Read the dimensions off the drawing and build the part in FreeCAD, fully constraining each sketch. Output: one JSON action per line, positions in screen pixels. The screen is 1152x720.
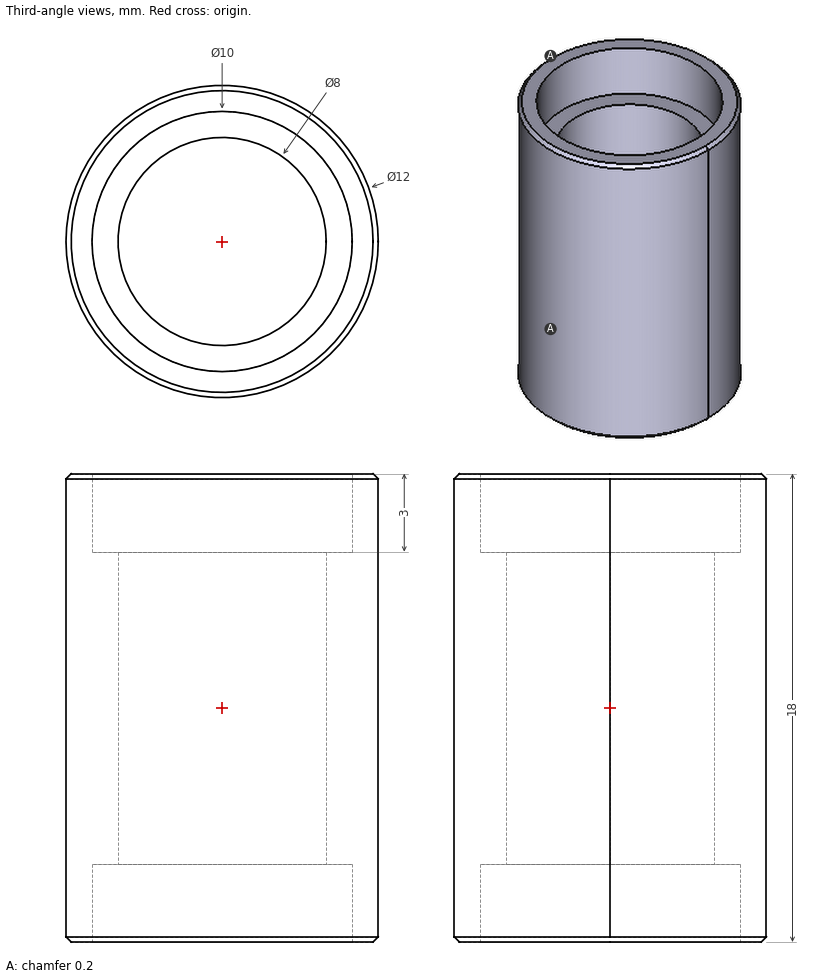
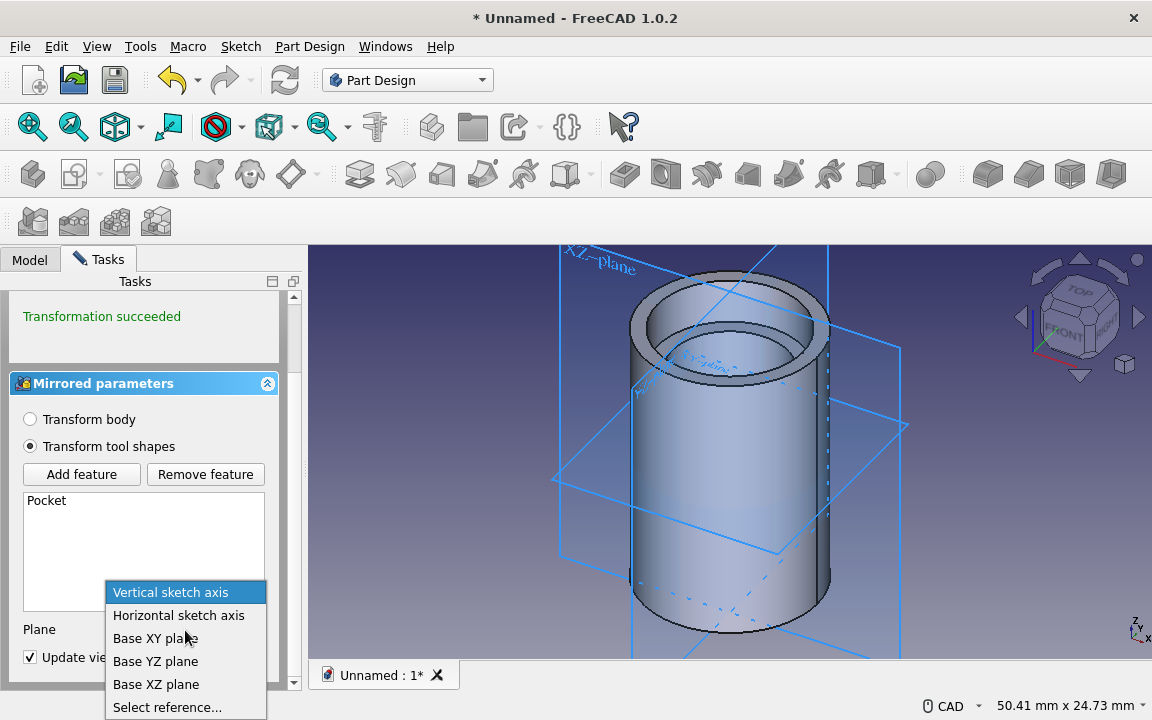
{"action": "left_click", "coordinate": [184, 638]}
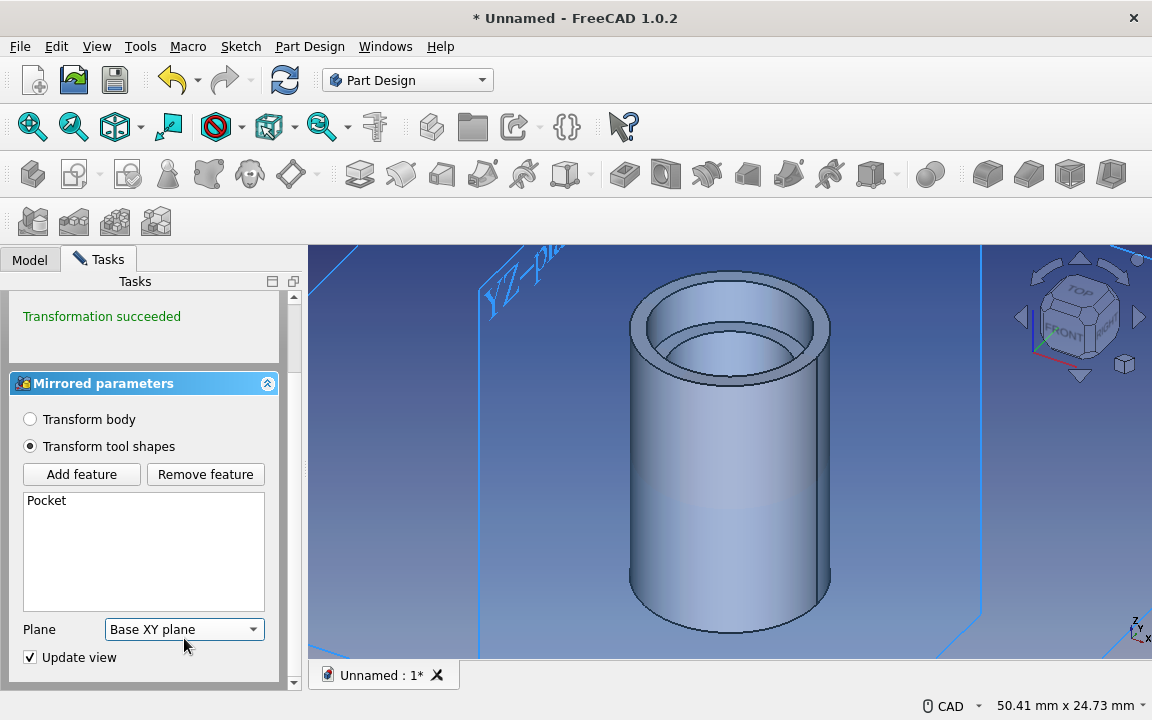
{"action": "scroll", "coordinate": [294, 490], "scroll_direction": "up", "scroll_amount": 3}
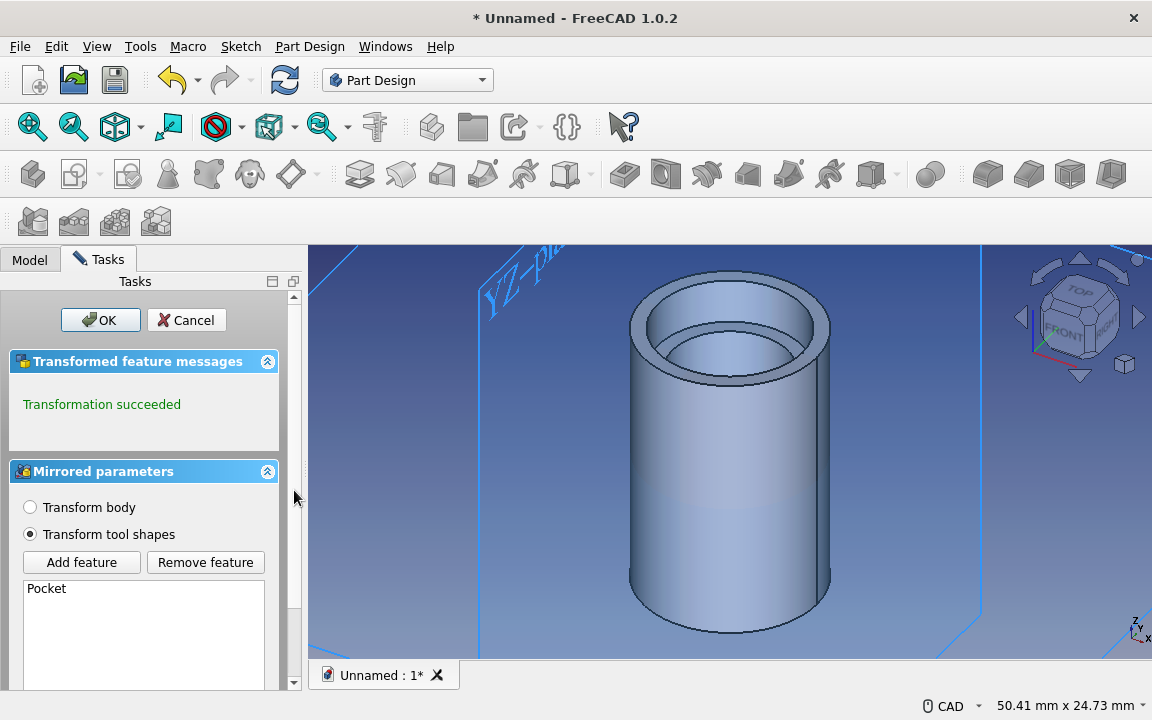
{"action": "left_click", "coordinate": [101, 320]}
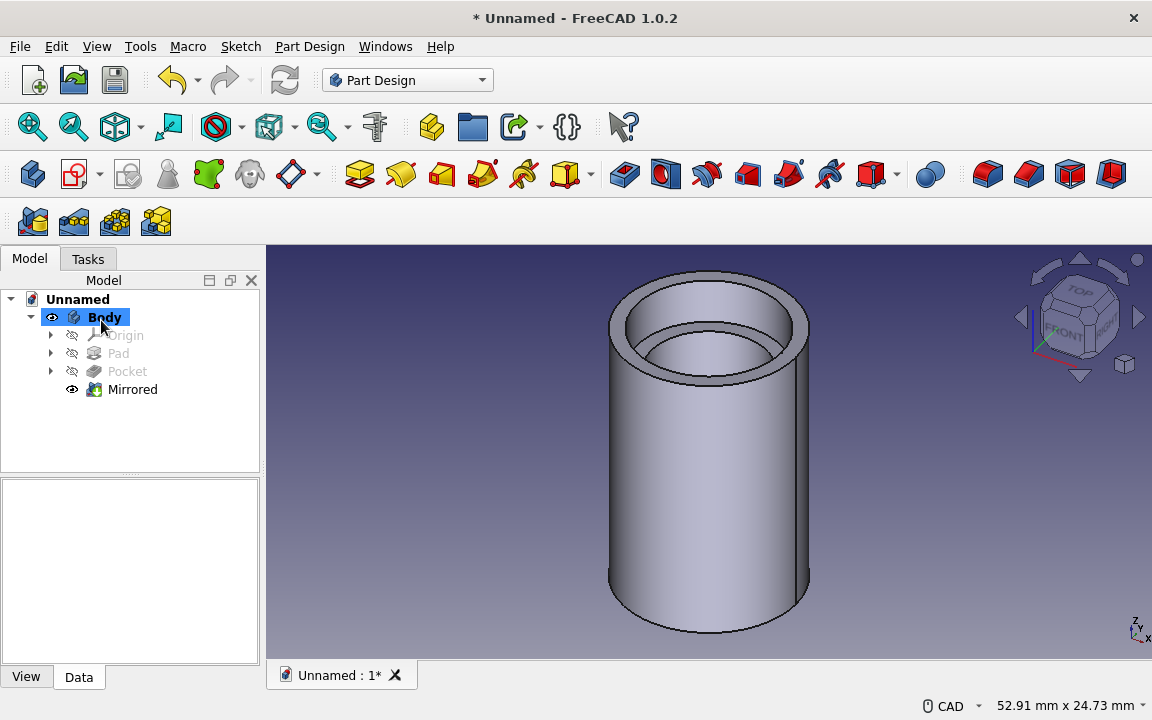
{"action": "left_click", "coordinate": [609, 334]}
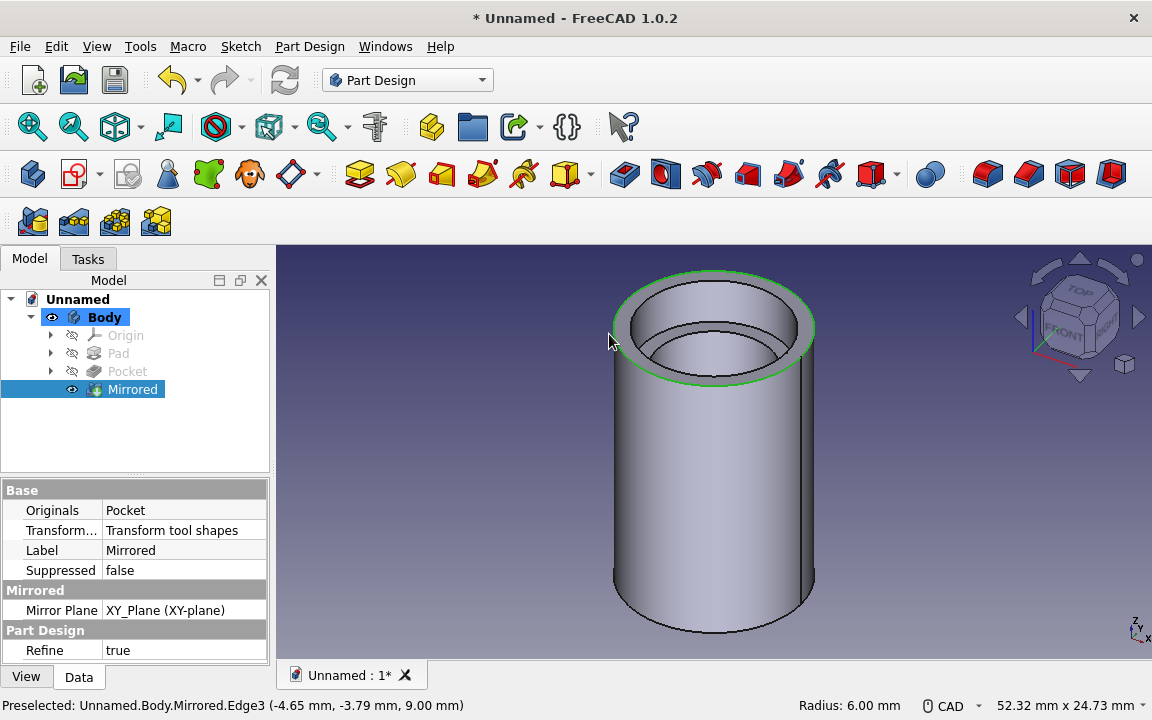
{"action": "key", "text": "0"}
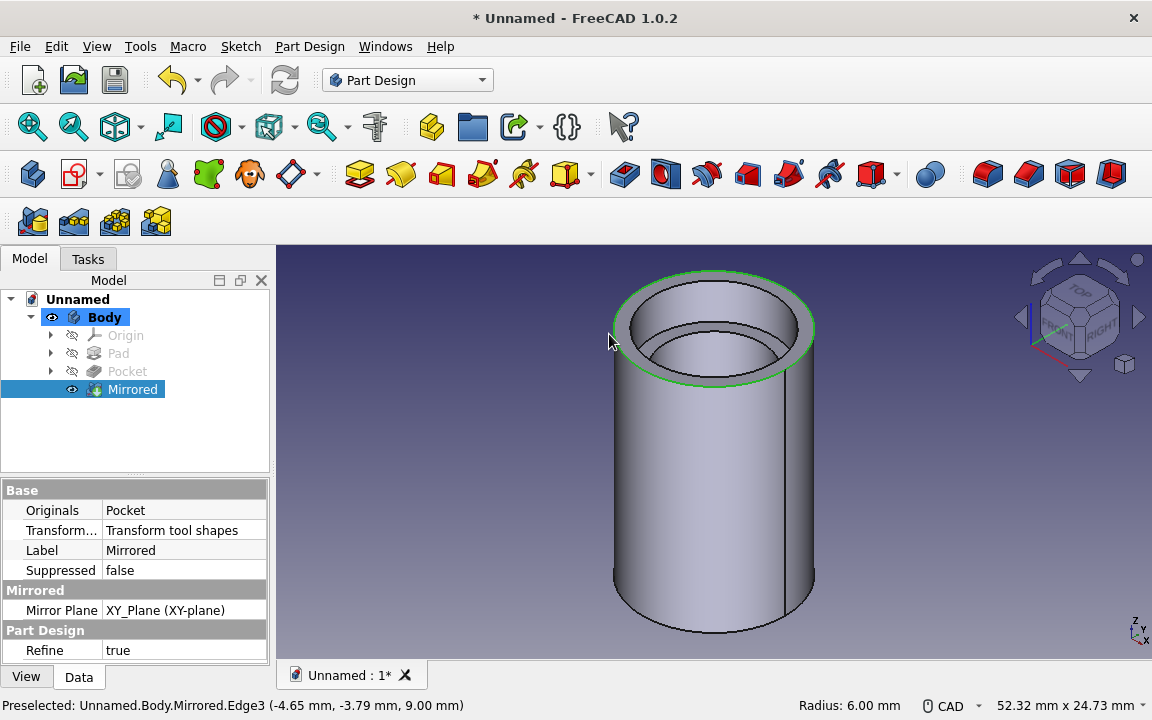
{"action": "left_click", "coordinate": [668, 626], "text": "ctrl"}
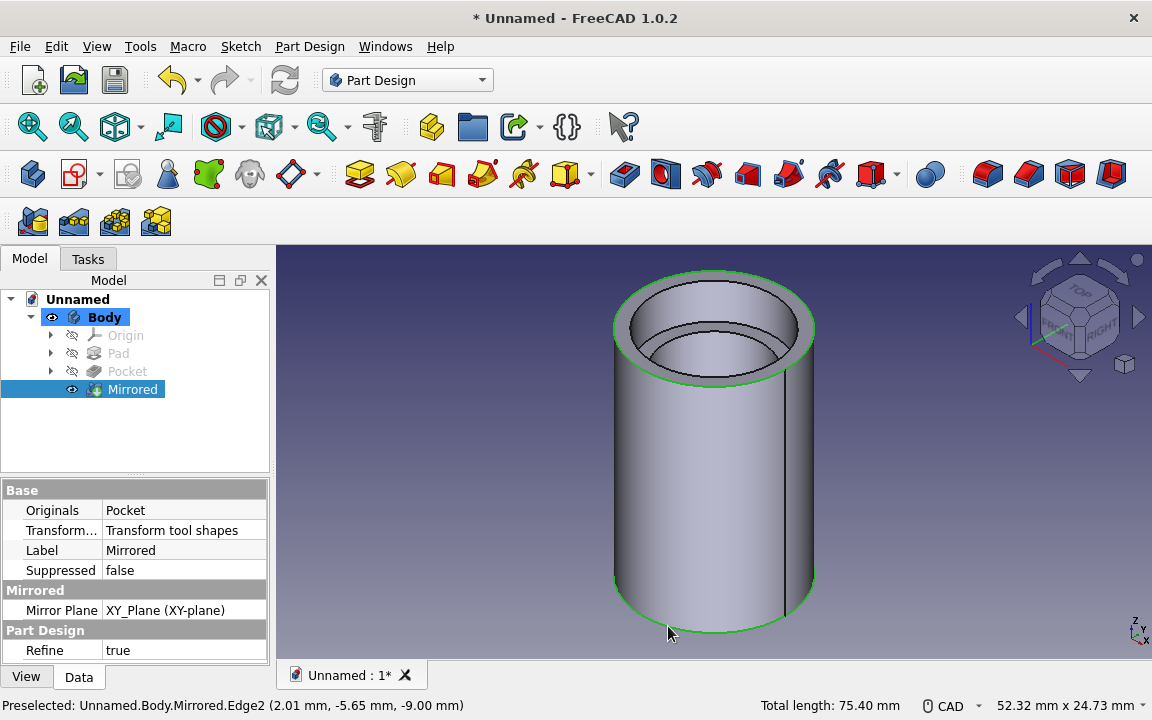
{"action": "left_click", "coordinate": [1029, 174]}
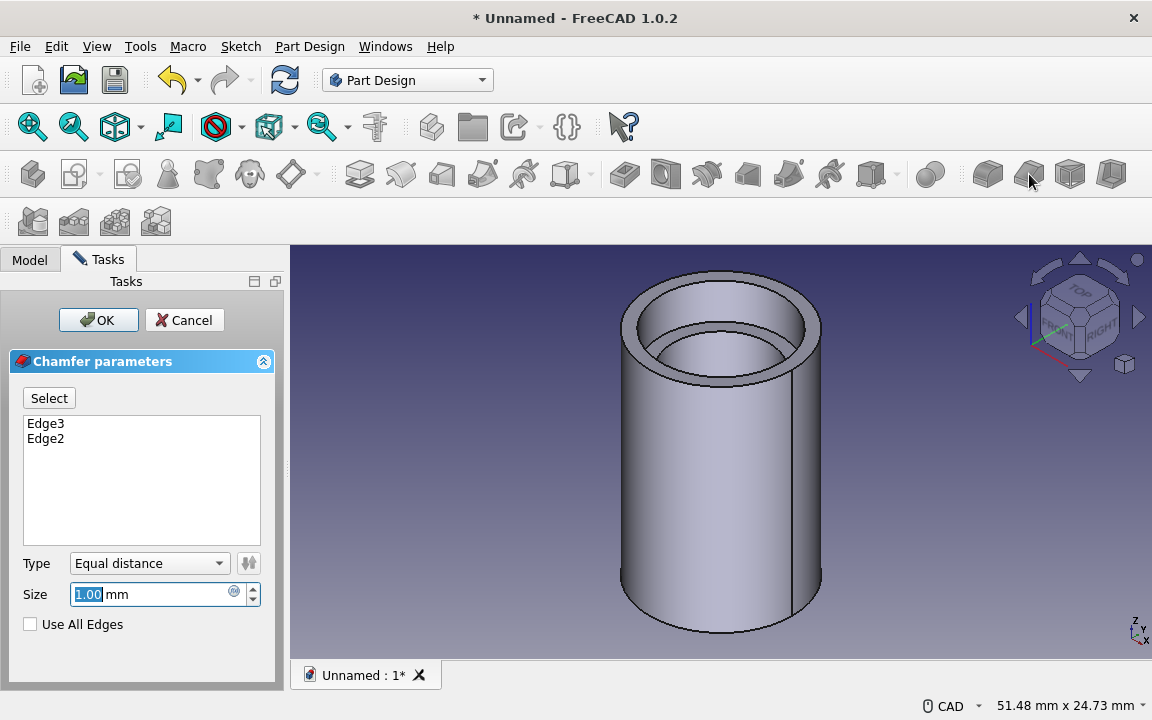
{"action": "type", "text": "0.2"}
{"action": "key", "text": "Tab"}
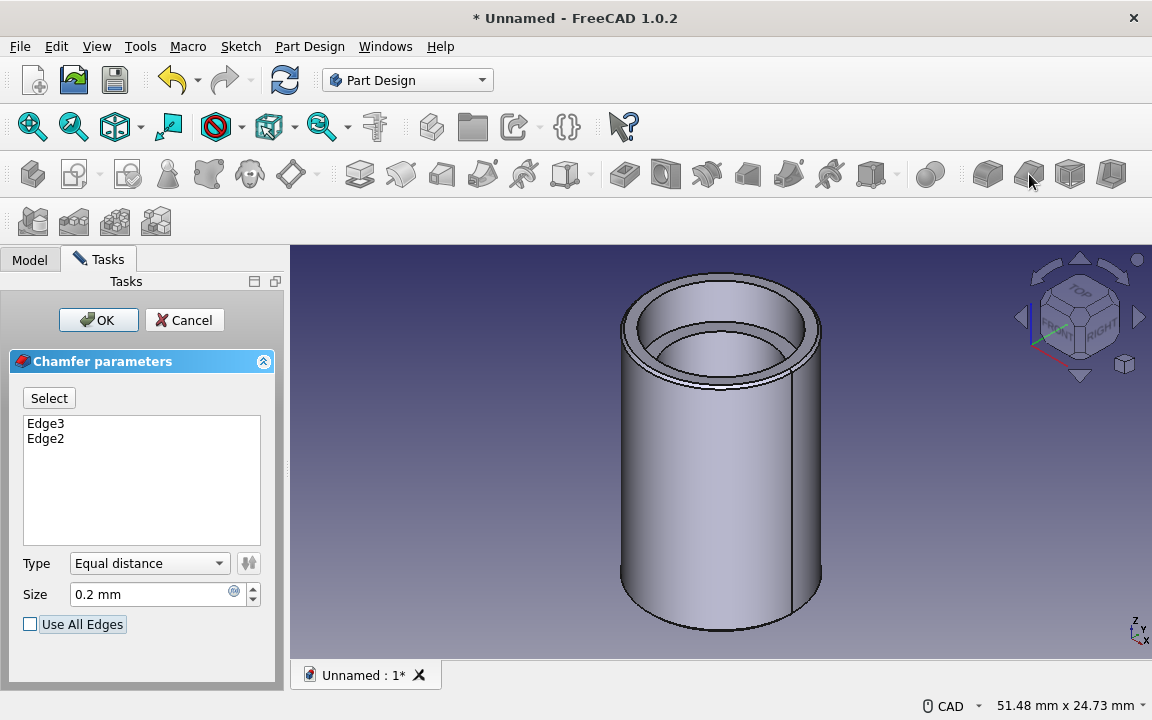
{"action": "left_click", "coordinate": [99, 320]}